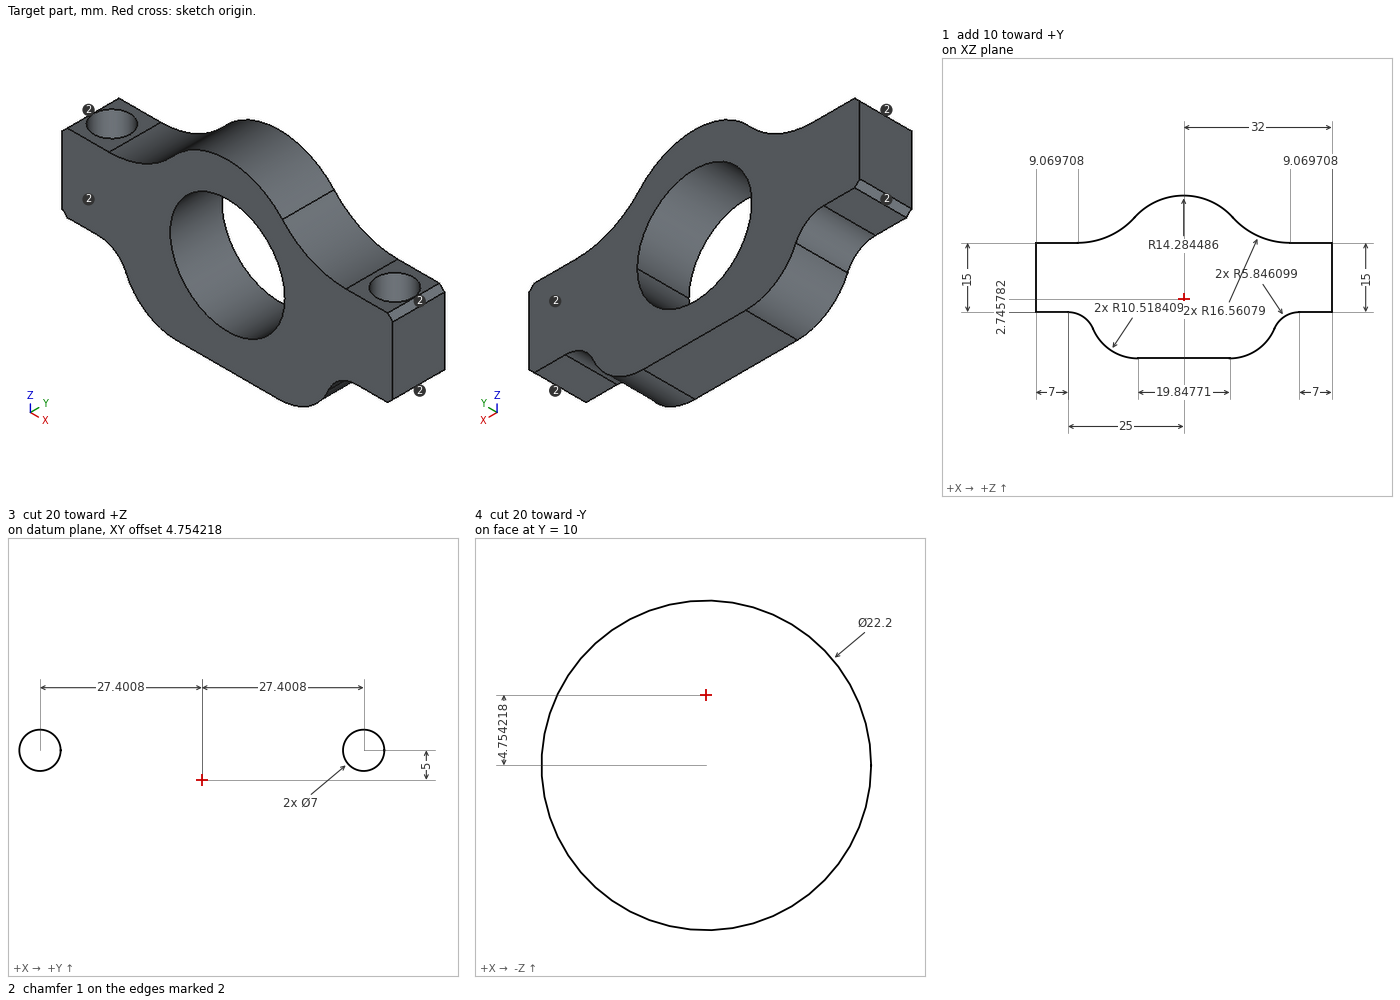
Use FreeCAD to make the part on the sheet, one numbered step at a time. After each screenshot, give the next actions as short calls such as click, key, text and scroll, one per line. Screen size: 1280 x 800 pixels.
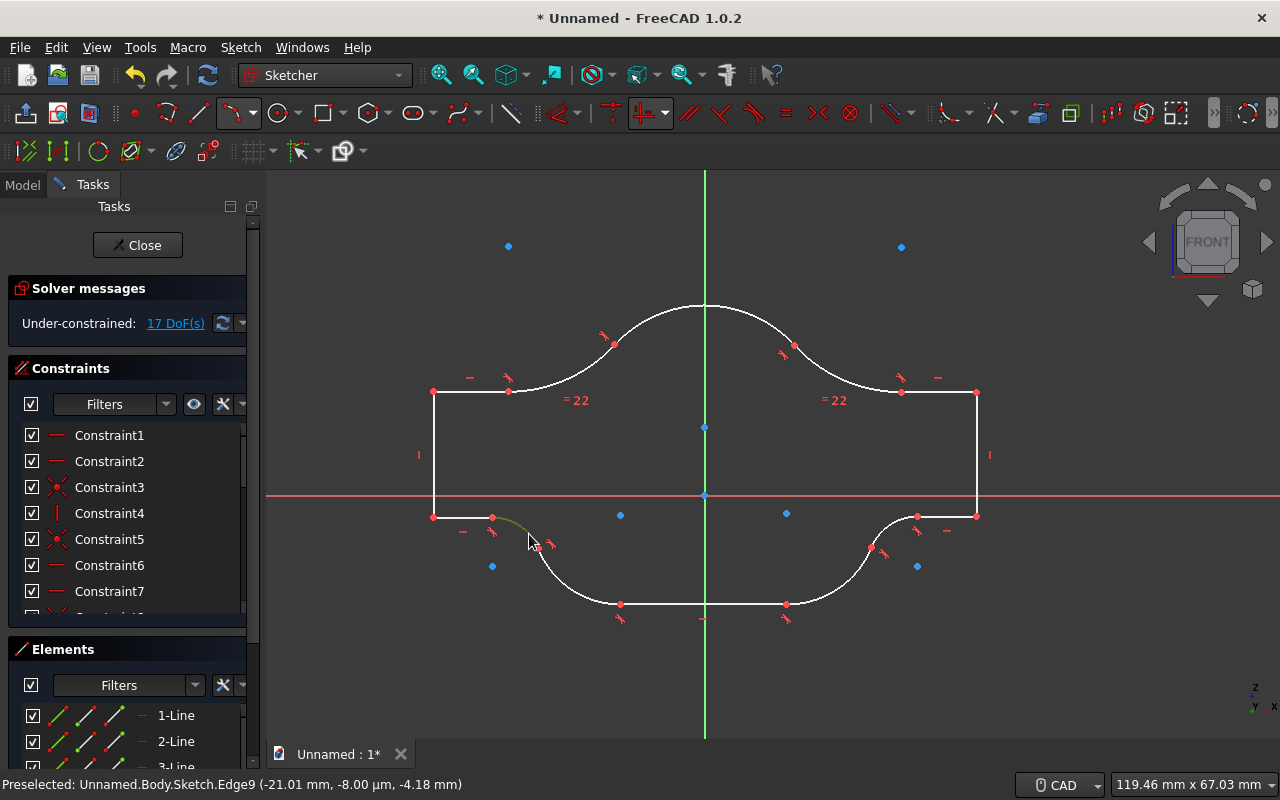
click(900, 520)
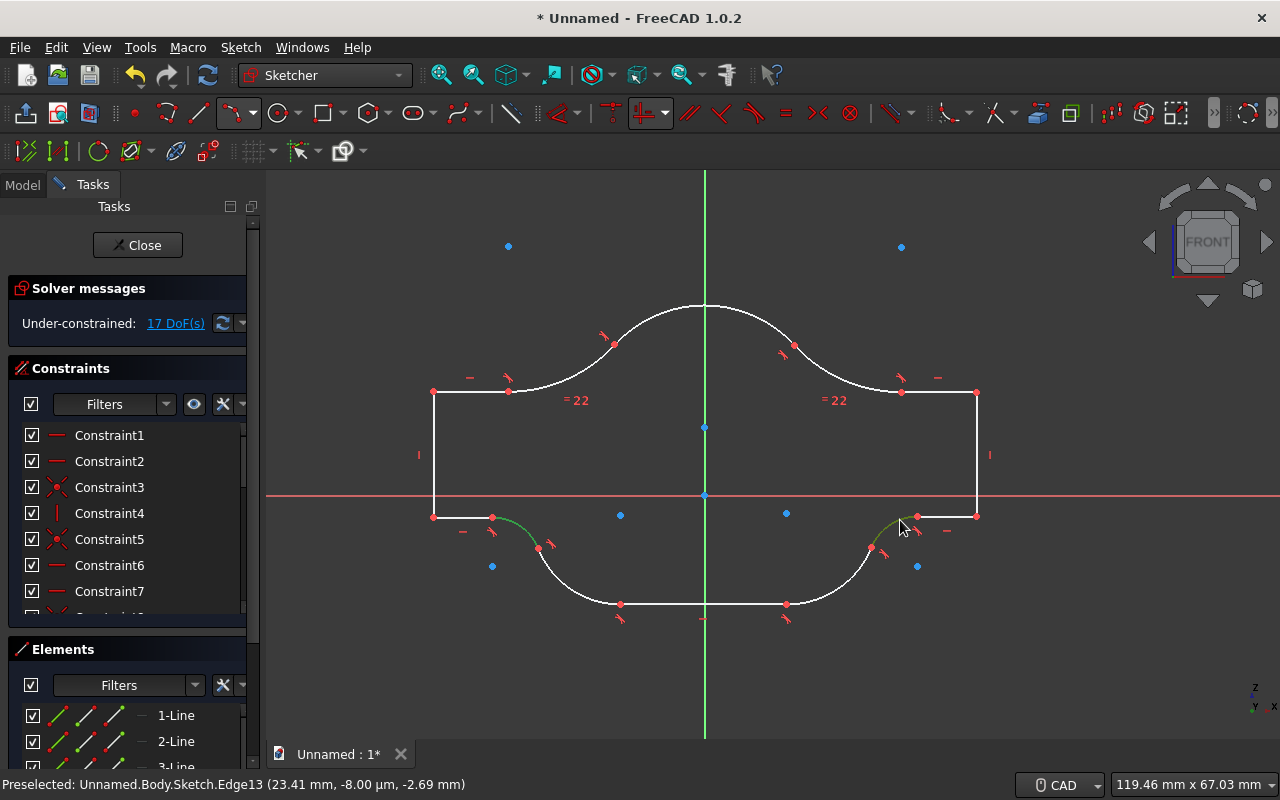
click(786, 114)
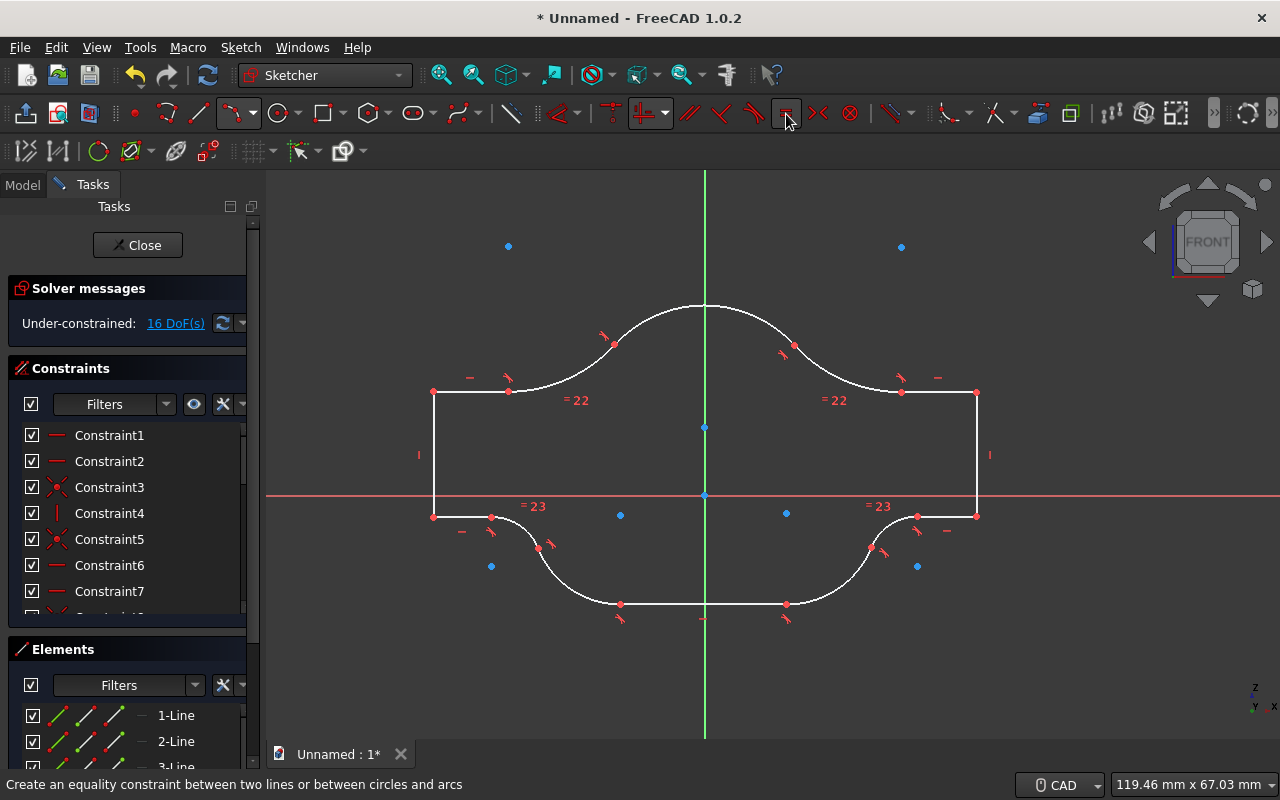
click(555, 575)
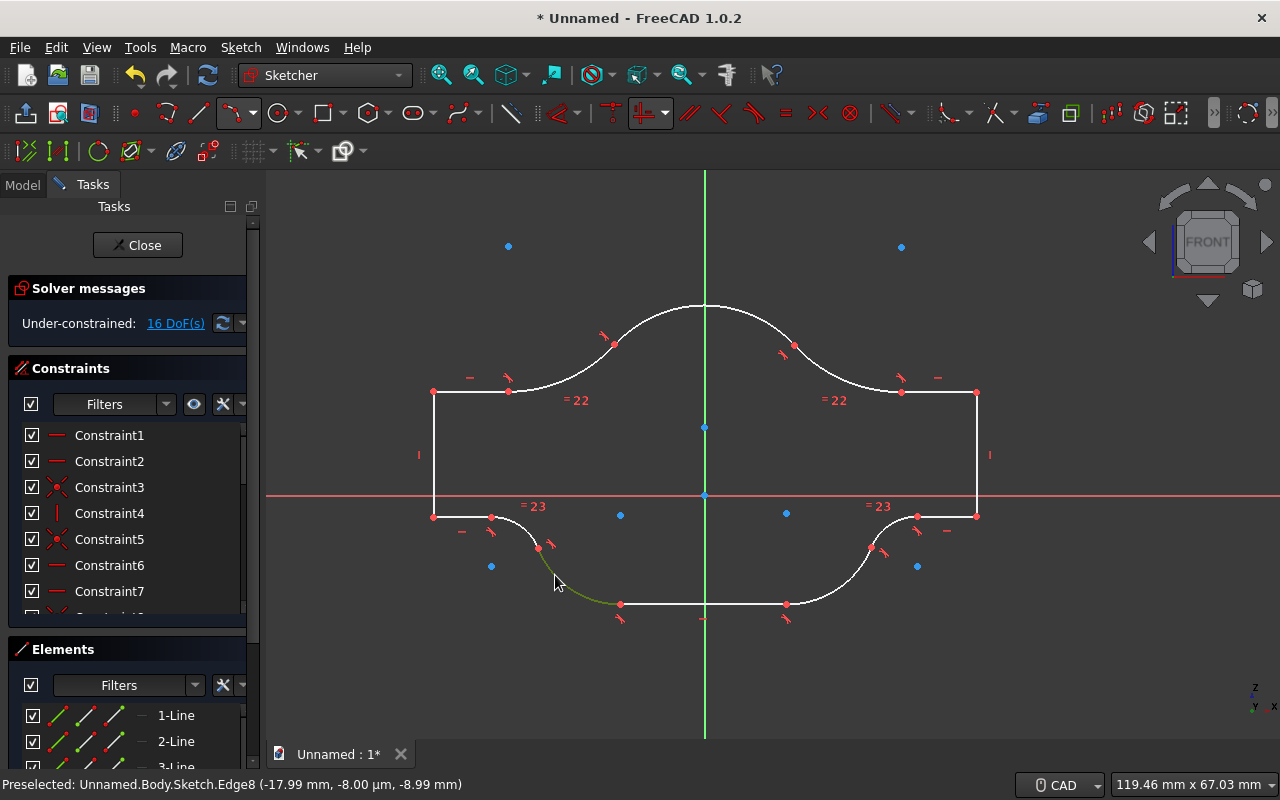
click(819, 599)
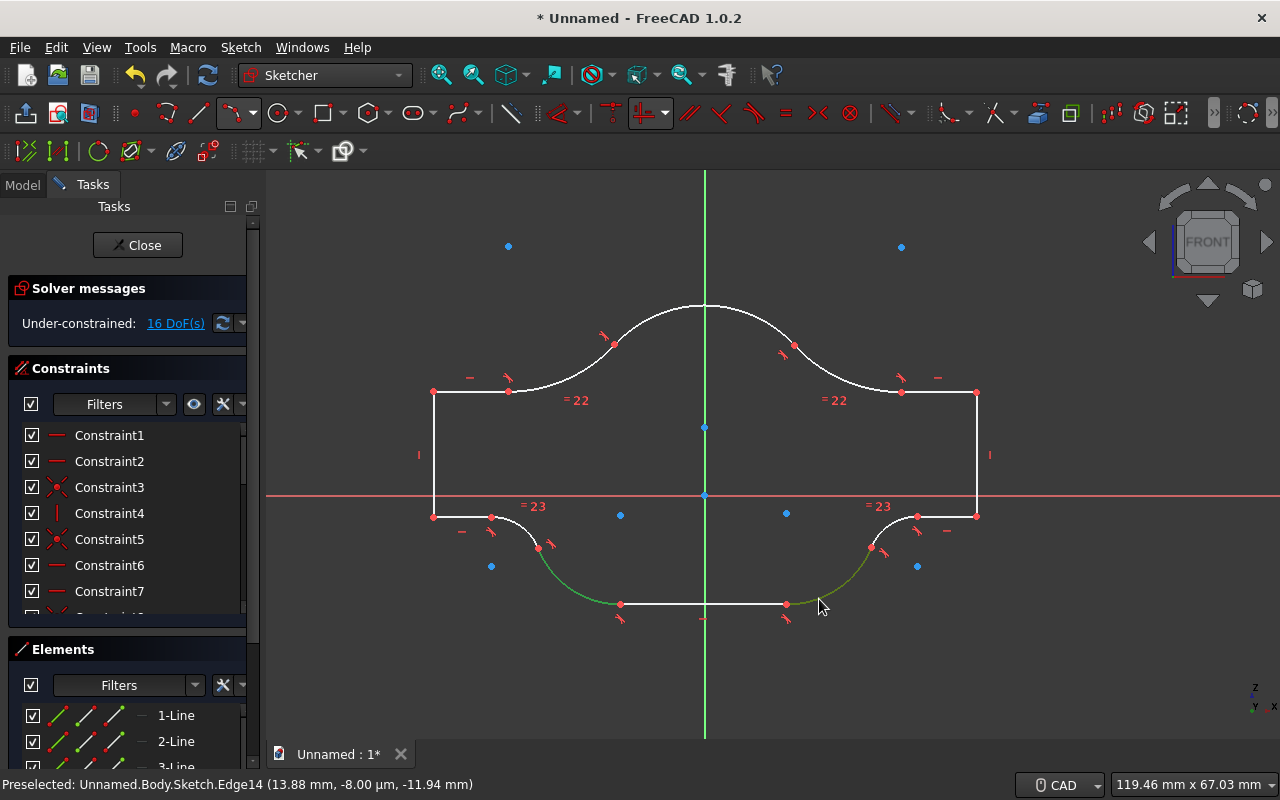
click(786, 114)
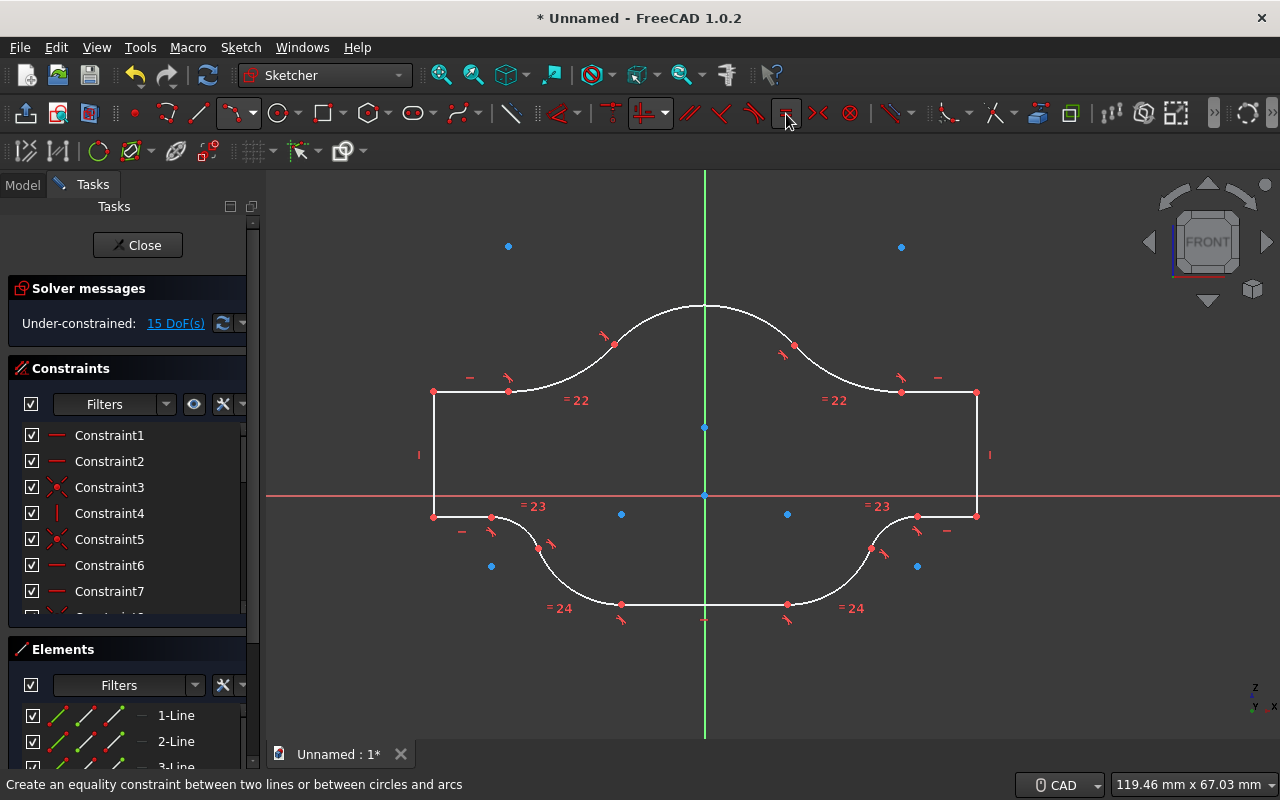
click(704, 427)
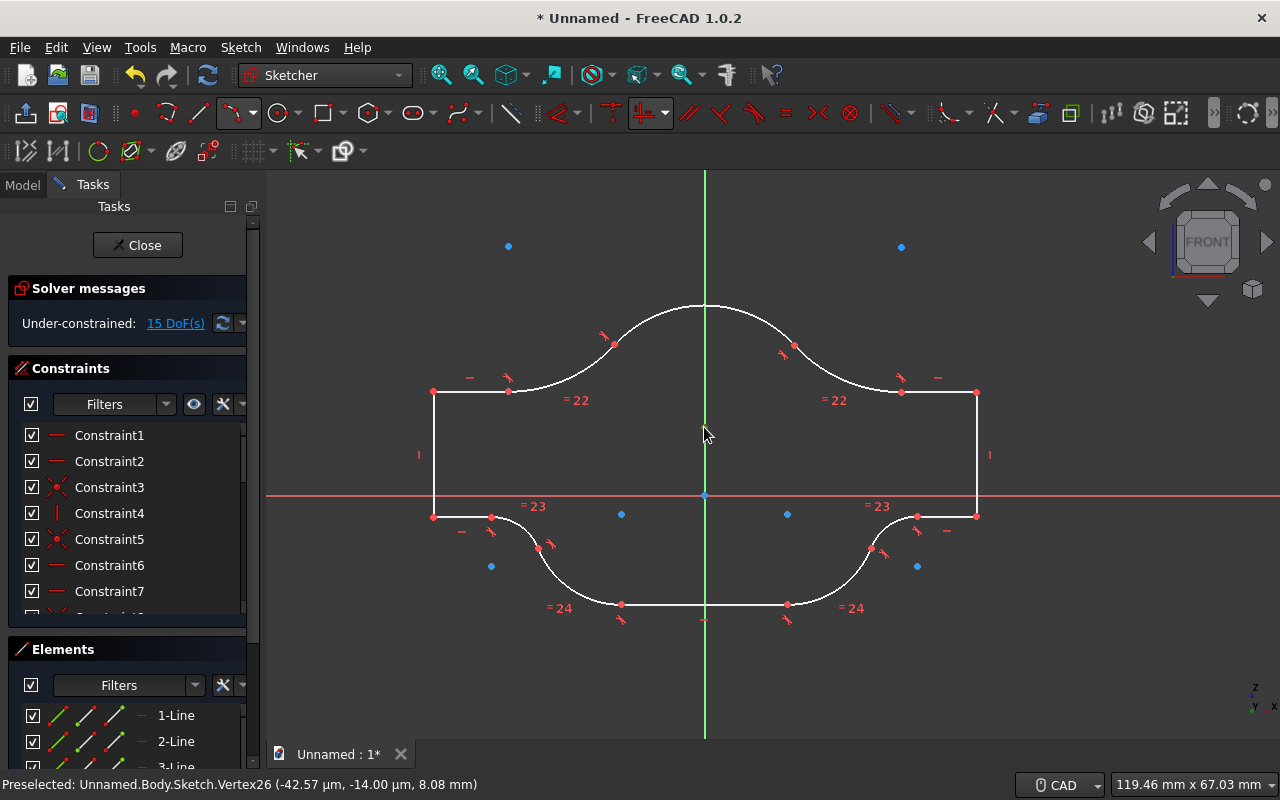
click(705, 674)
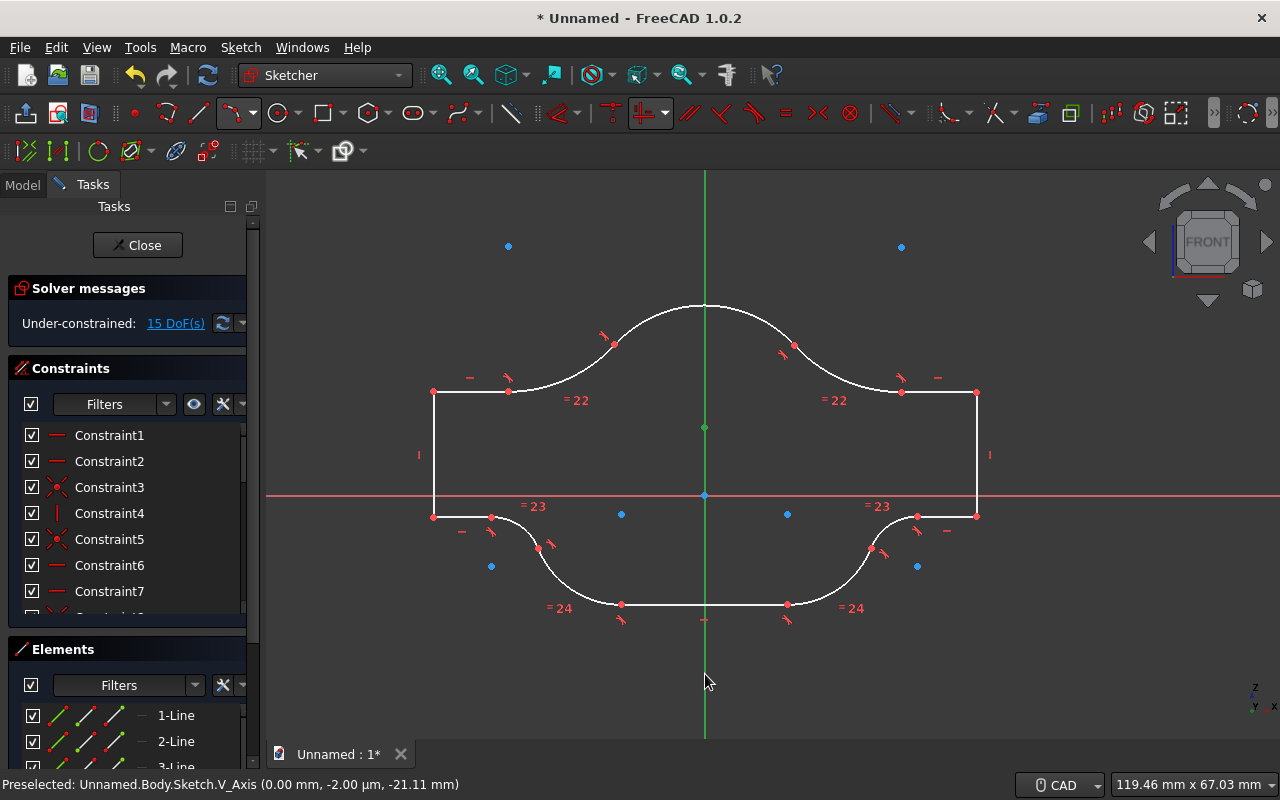
click(612, 114)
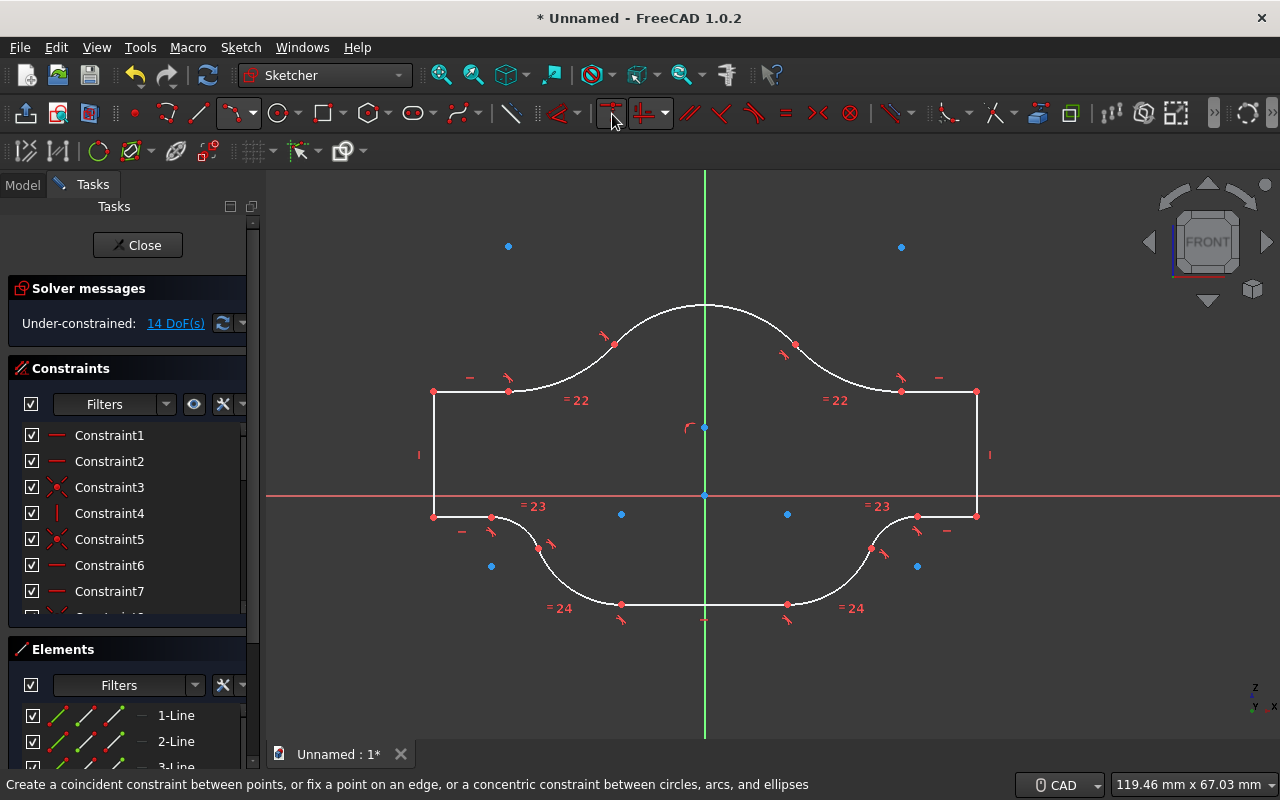
click(558, 114)